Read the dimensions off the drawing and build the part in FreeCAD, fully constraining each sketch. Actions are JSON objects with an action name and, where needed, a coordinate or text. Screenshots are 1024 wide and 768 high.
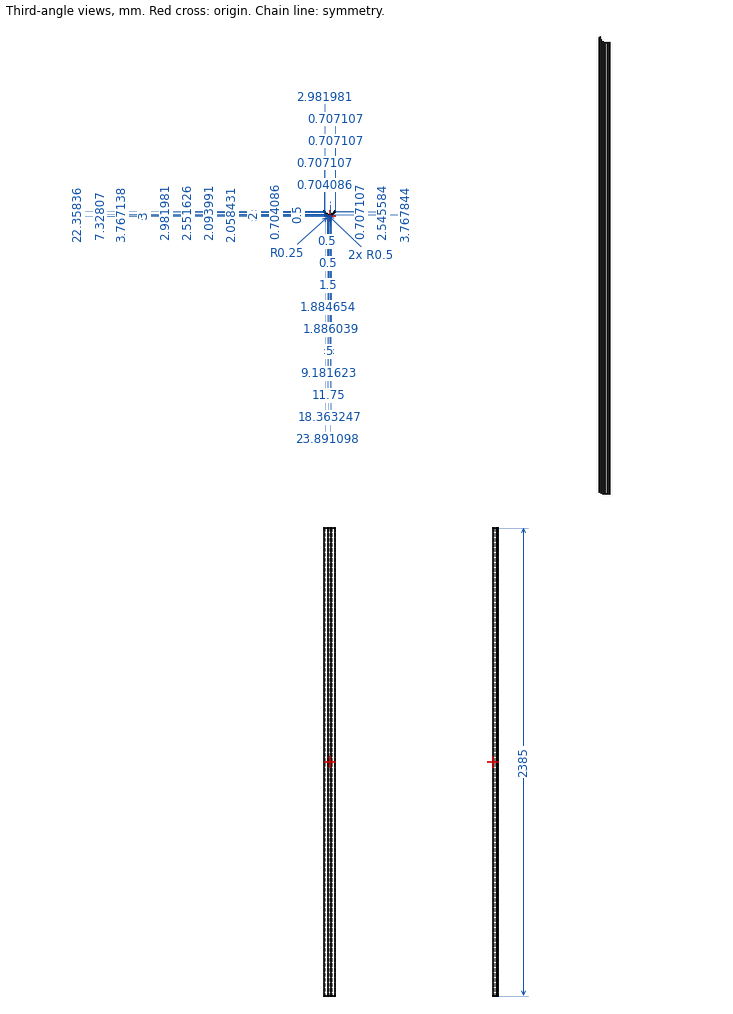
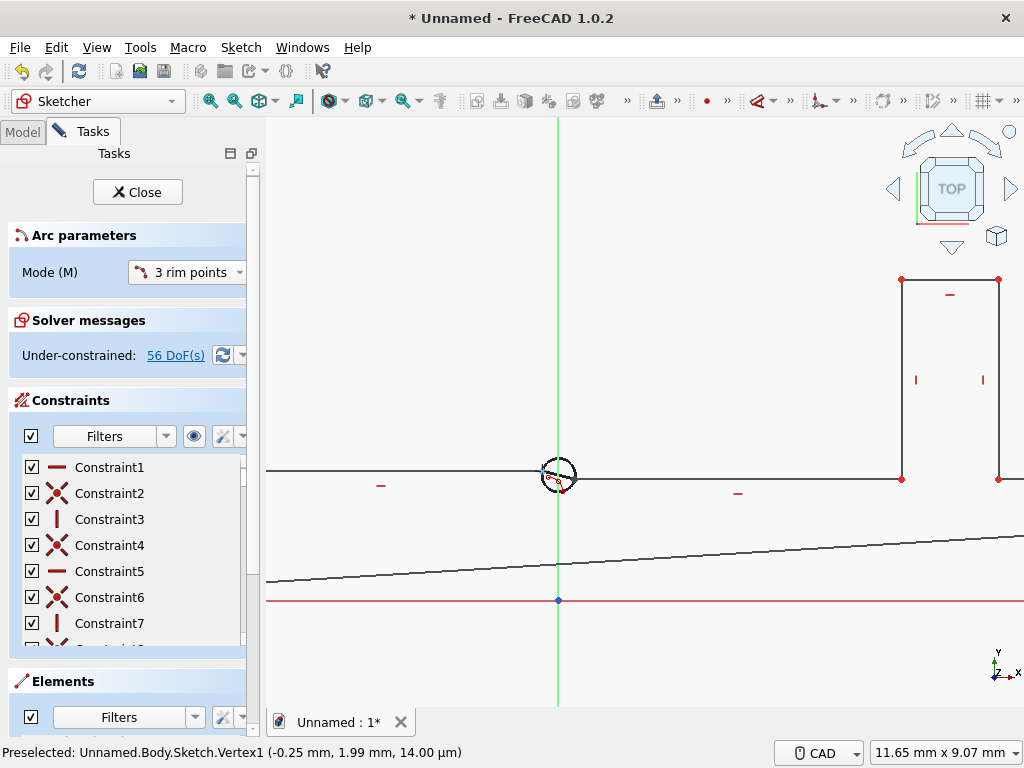
{"action": "scroll", "coordinate": [549, 484], "scroll_direction": "up", "scroll_amount": 3}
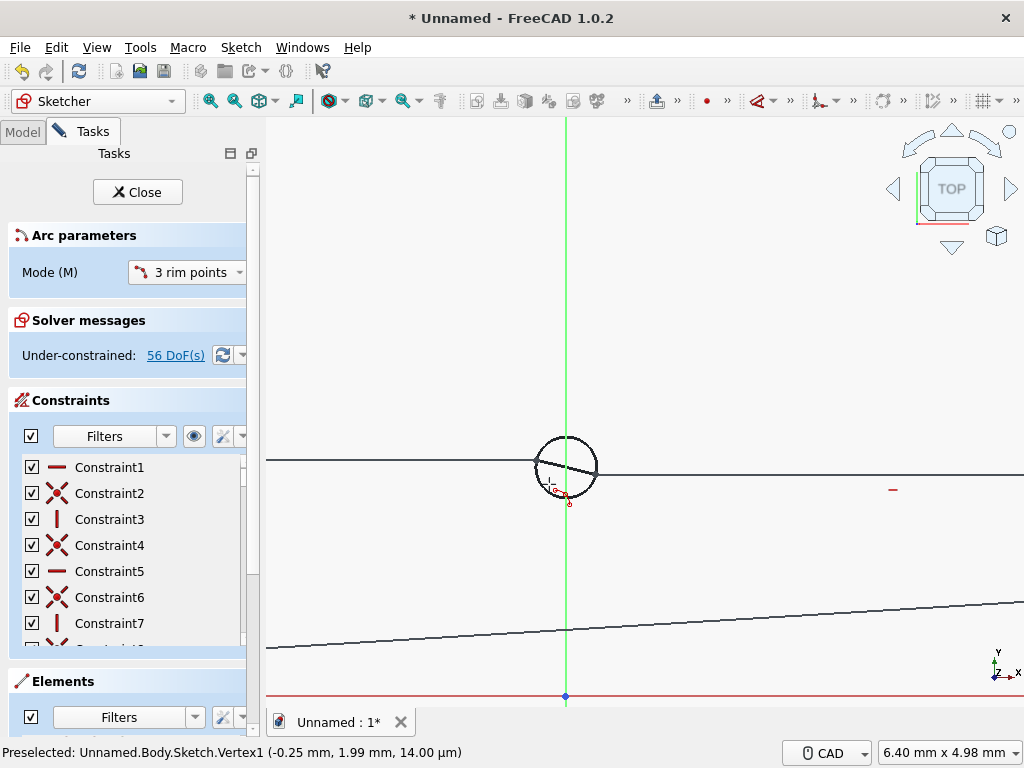
{"action": "left_click", "coordinate": [549, 483]}
{"action": "key", "text": "Escape"}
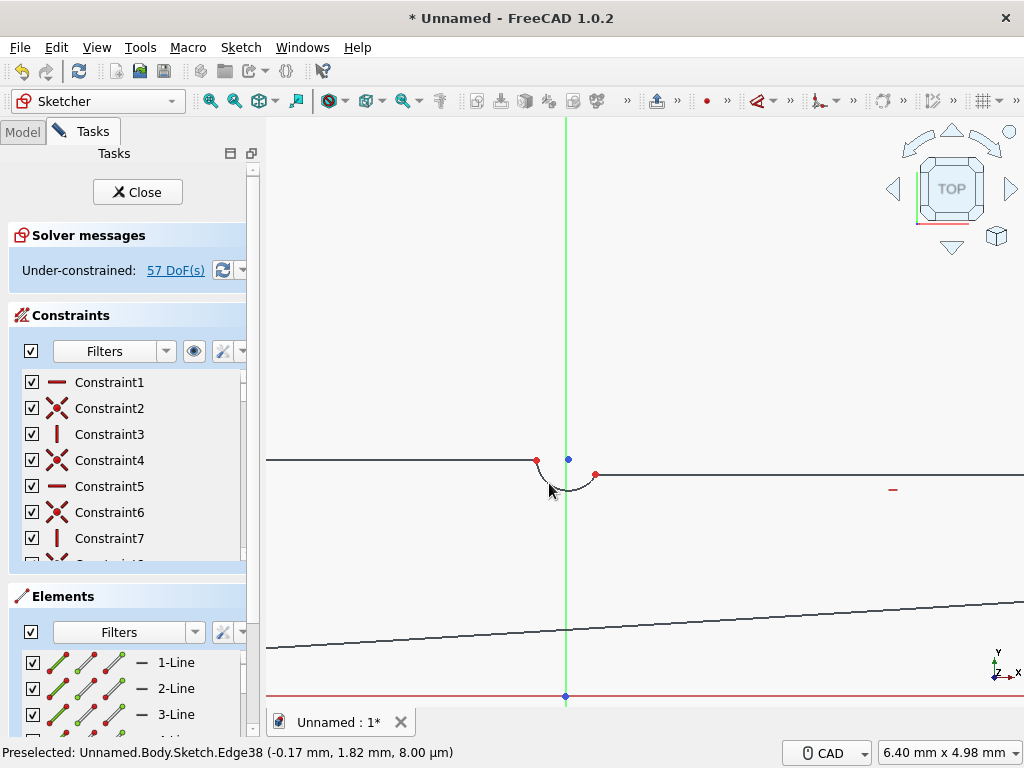
{"action": "scroll", "coordinate": [577, 479], "scroll_direction": "down", "scroll_amount": 14}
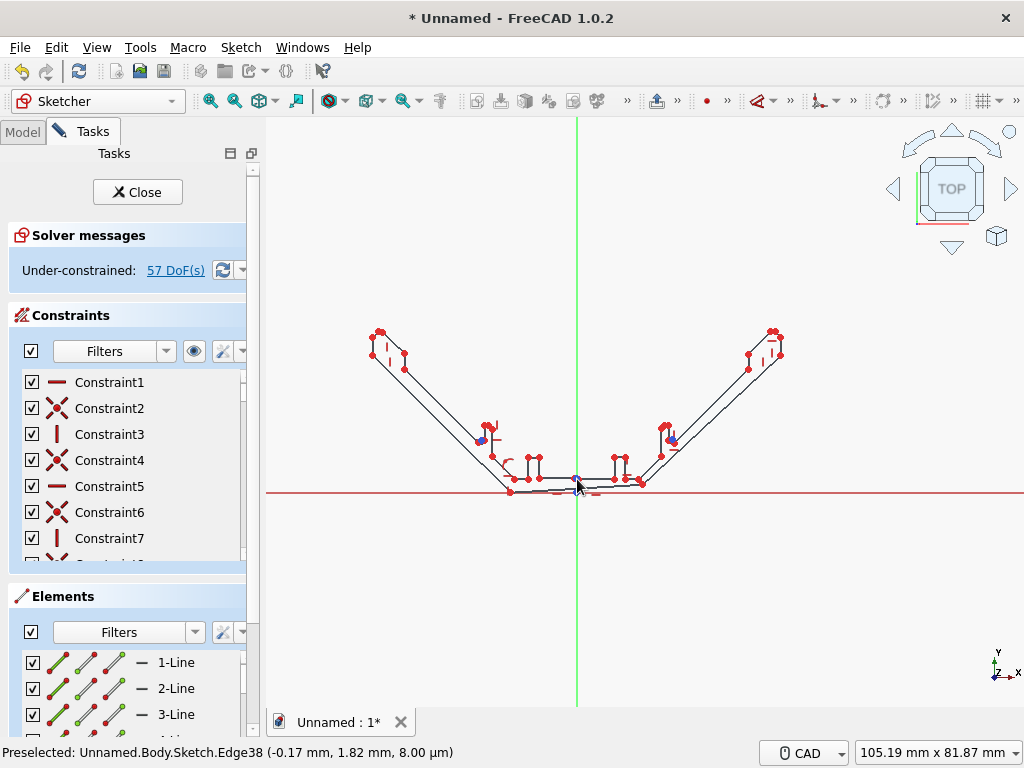
{"action": "scroll", "coordinate": [485, 430], "scroll_direction": "up", "scroll_amount": 6}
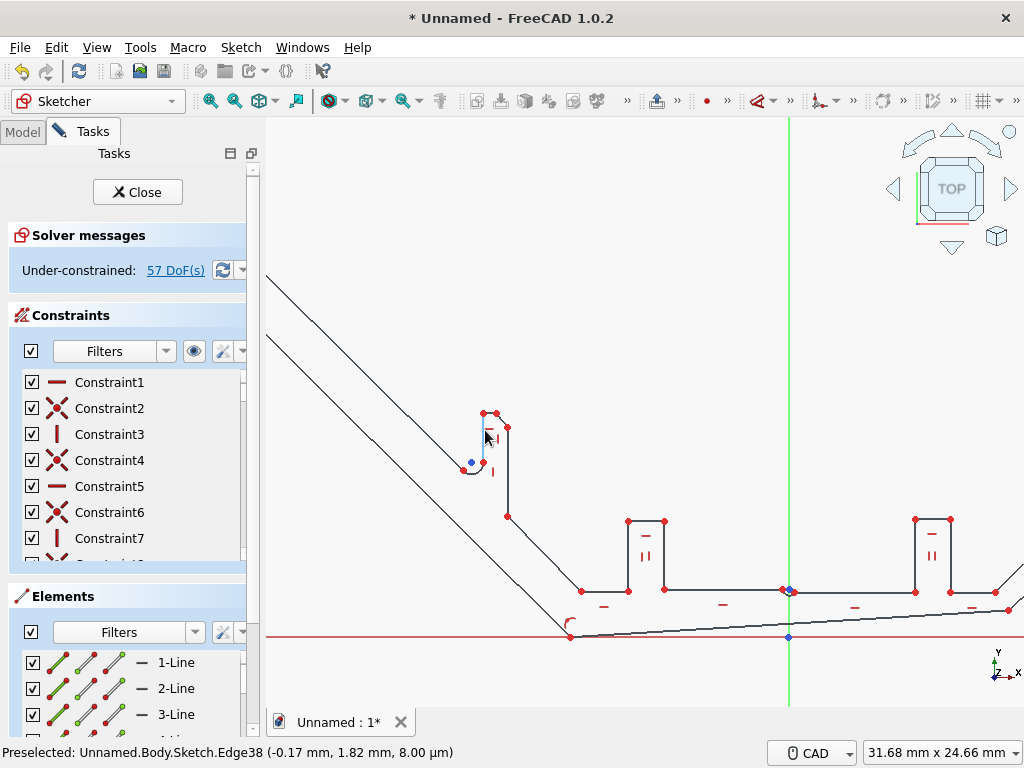
{"action": "left_click", "coordinate": [483, 428]}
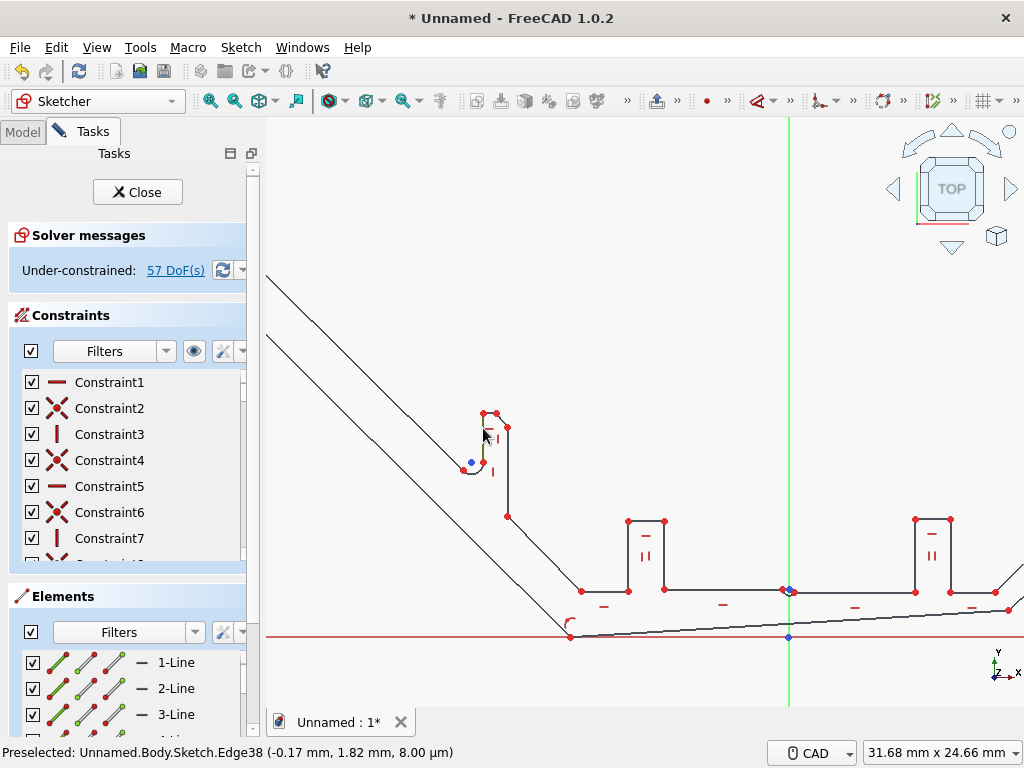
{"action": "left_click", "coordinate": [476, 474]}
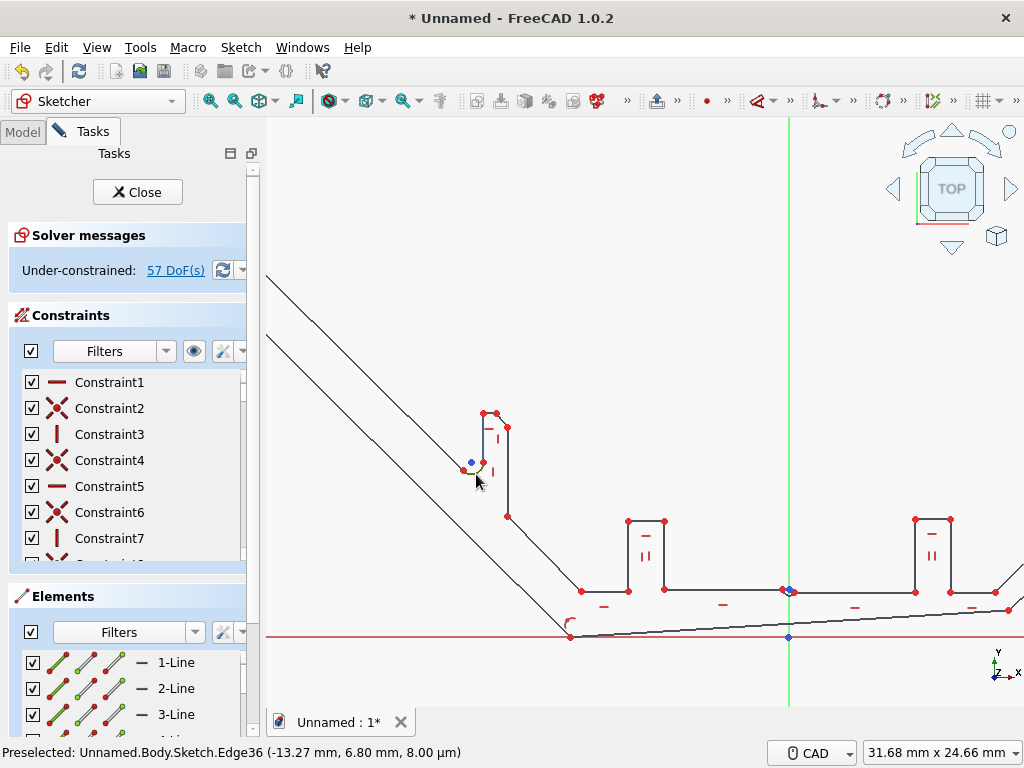
{"action": "key", "text": "t"}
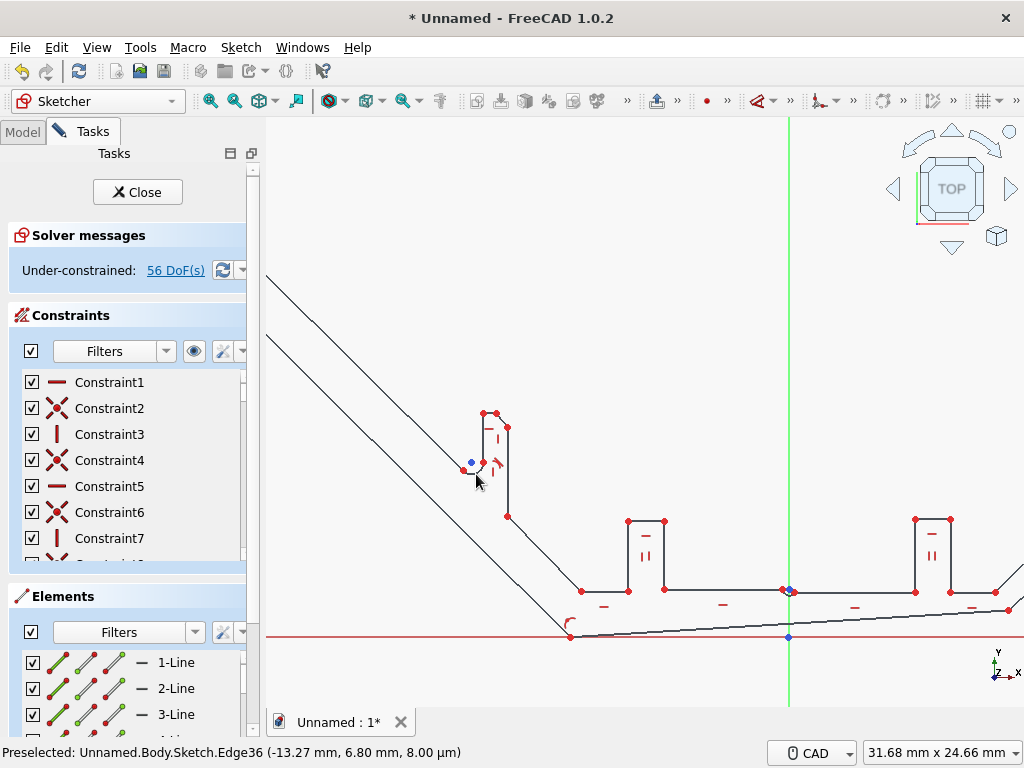
{"action": "scroll", "coordinate": [485, 430], "scroll_direction": "down", "scroll_amount": 6}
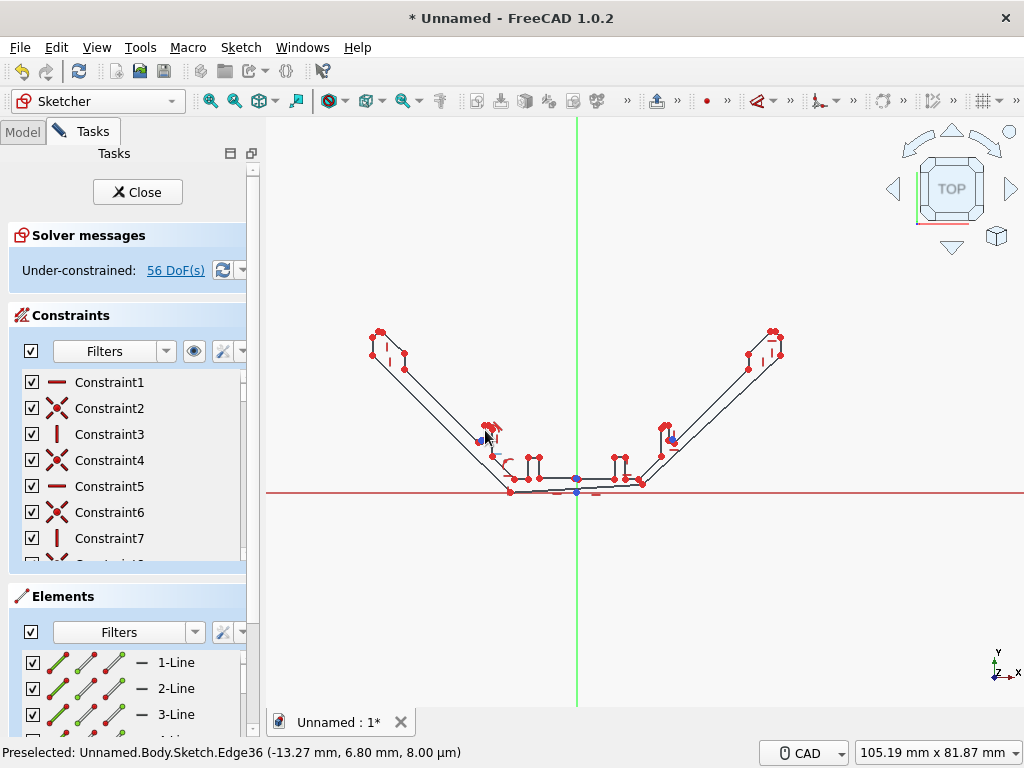
{"action": "left_click", "coordinate": [457, 421]}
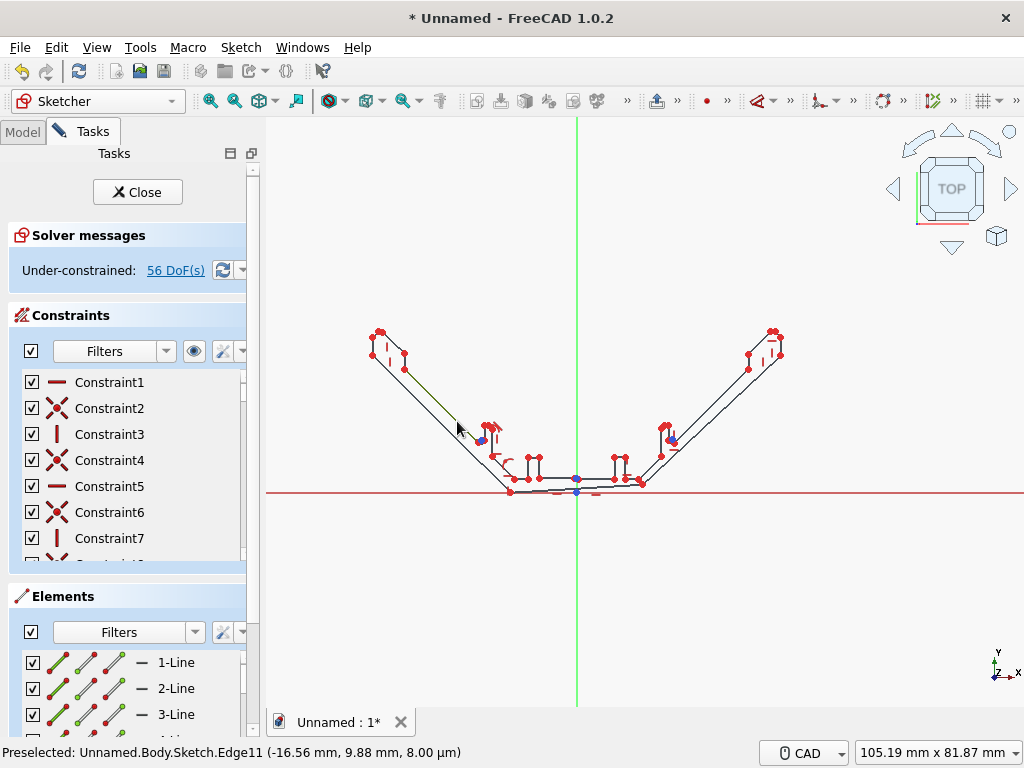
{"action": "scroll", "coordinate": [483, 443], "scroll_direction": "up", "scroll_amount": 7}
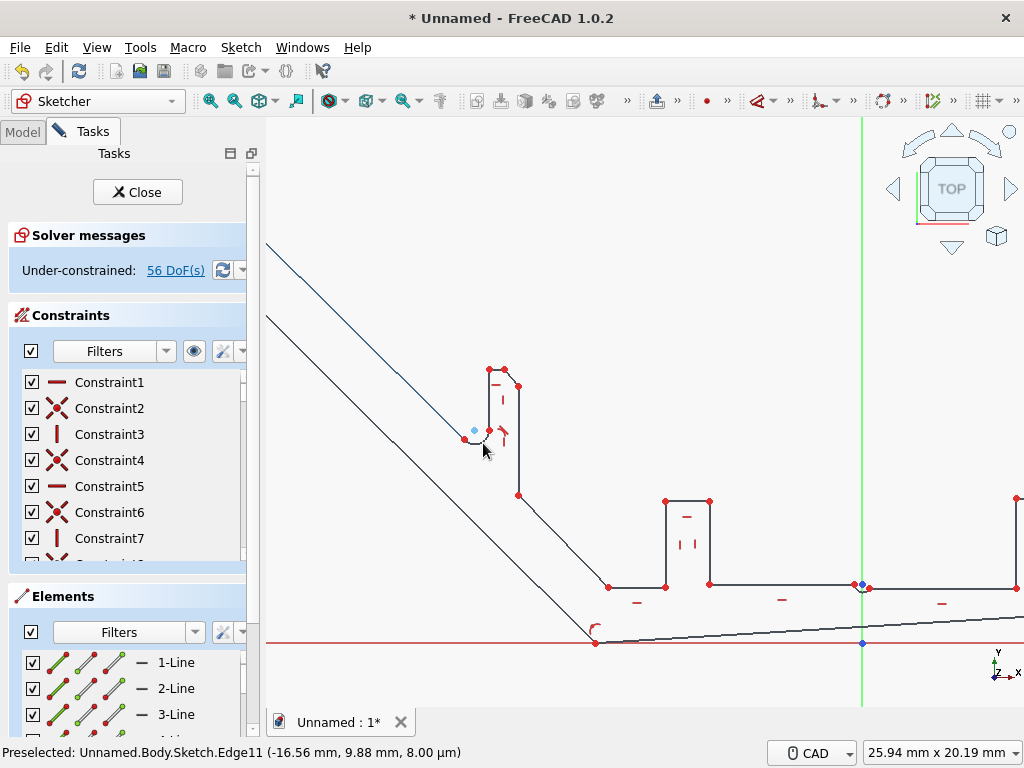
{"action": "left_click", "coordinate": [480, 443]}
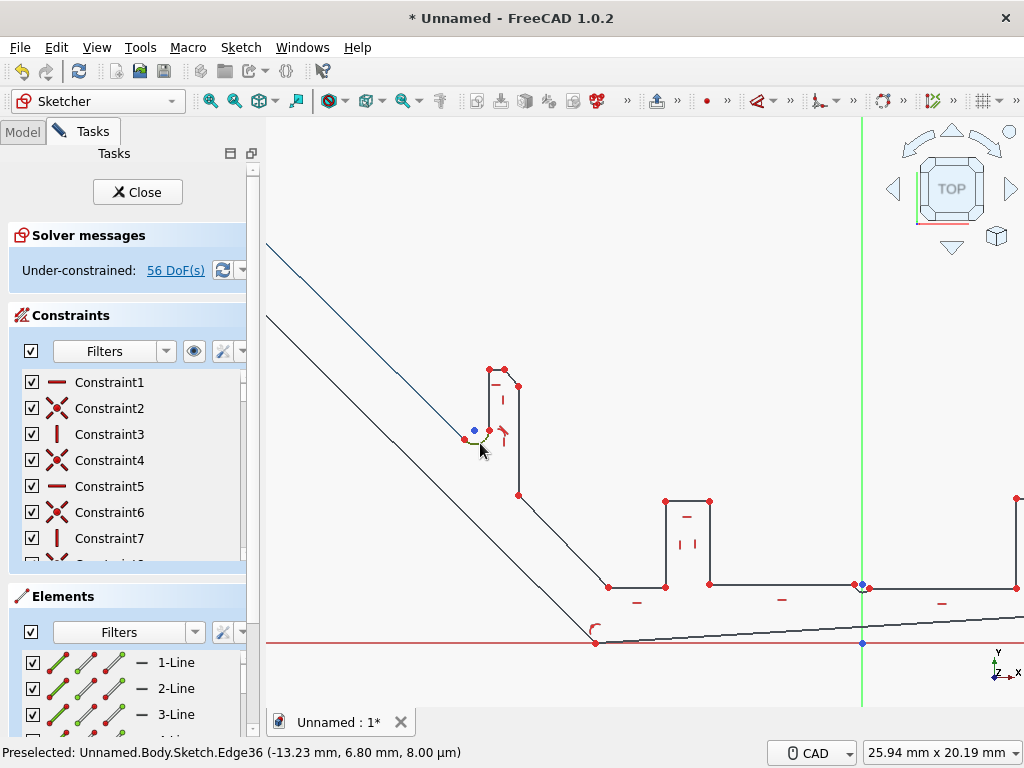
{"action": "key", "text": "t"}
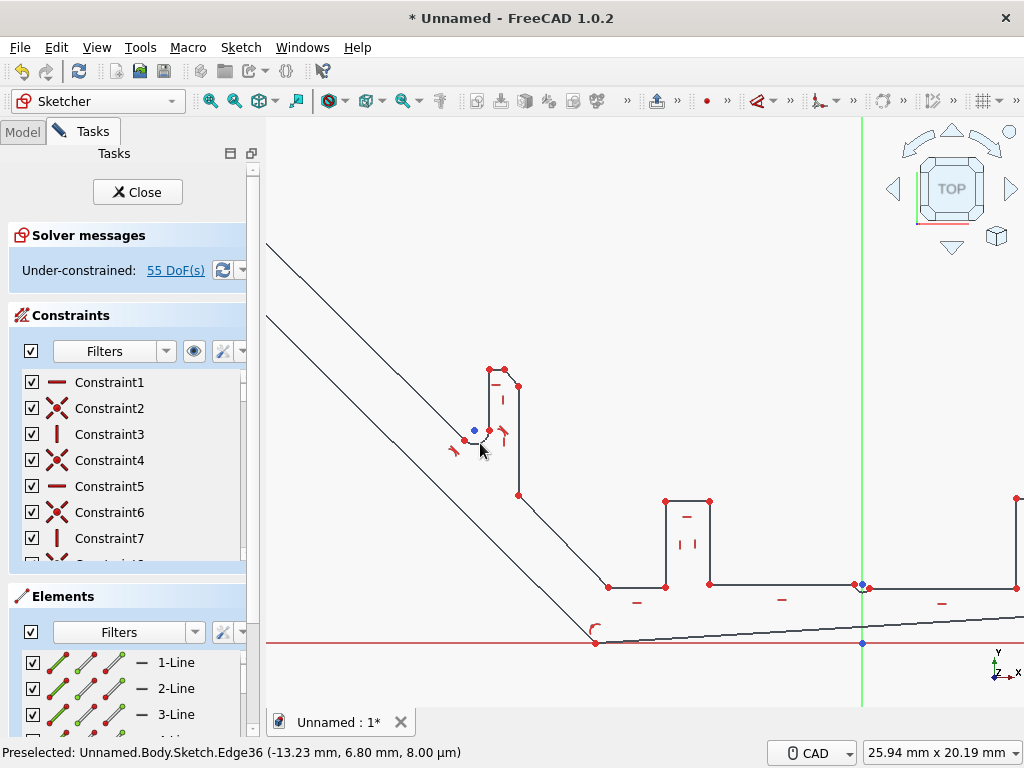
{"action": "scroll", "coordinate": [483, 443], "scroll_direction": "down", "scroll_amount": 7}